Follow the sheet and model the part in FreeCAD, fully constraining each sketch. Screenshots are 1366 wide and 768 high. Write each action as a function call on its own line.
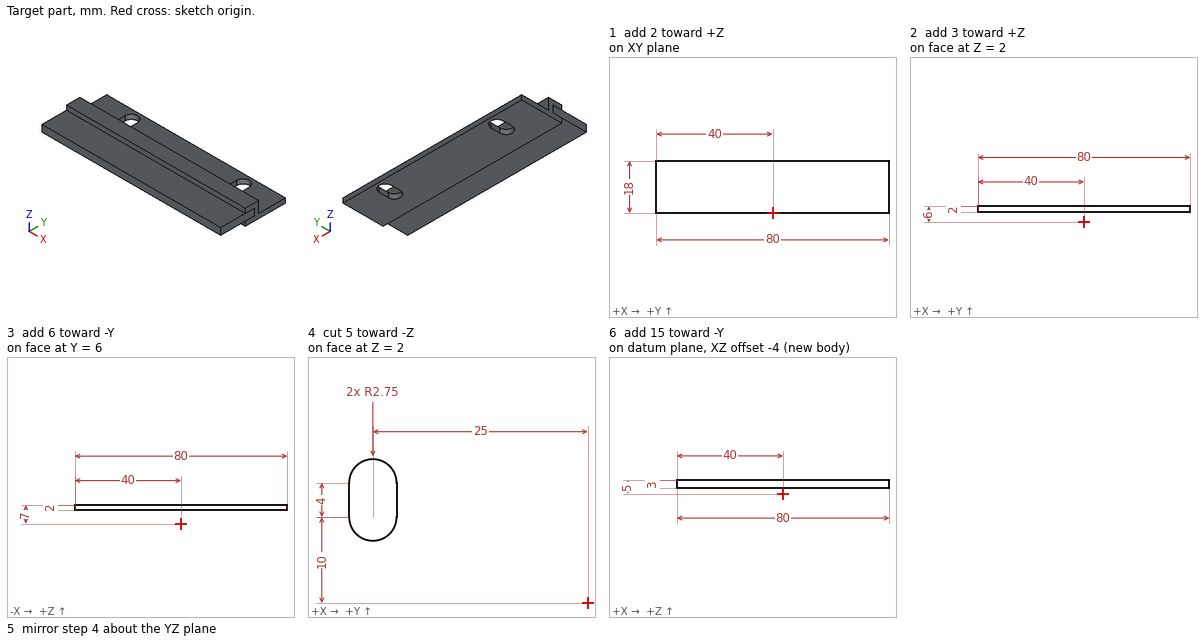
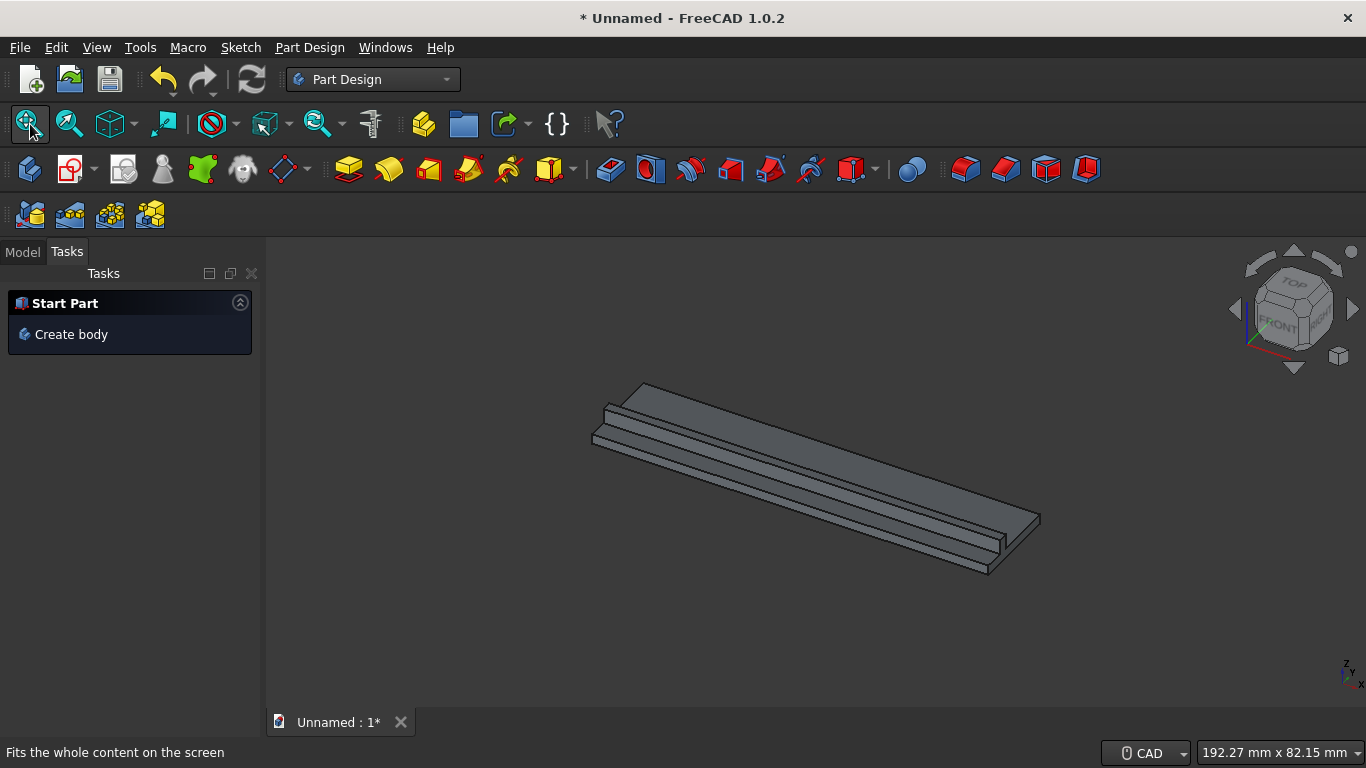
key(4)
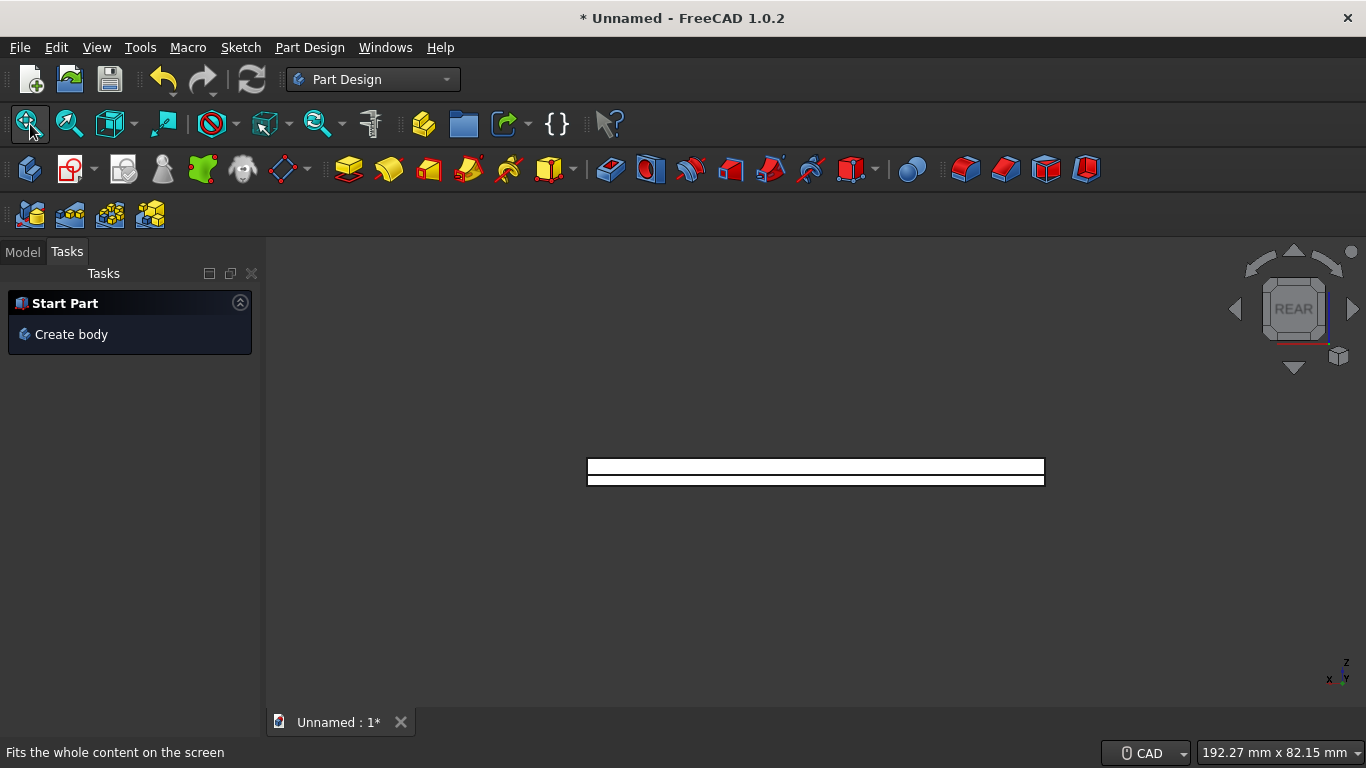
key(v)
key(f)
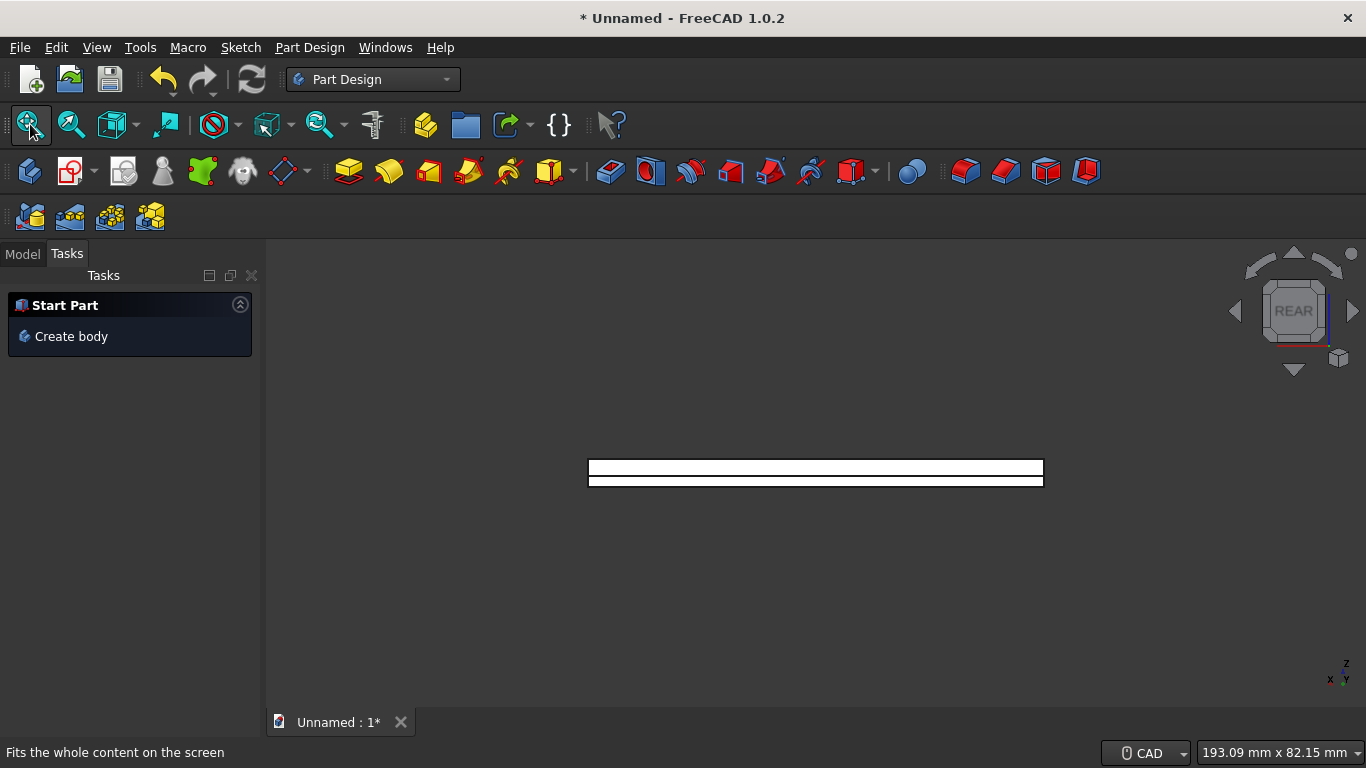
click(621, 466)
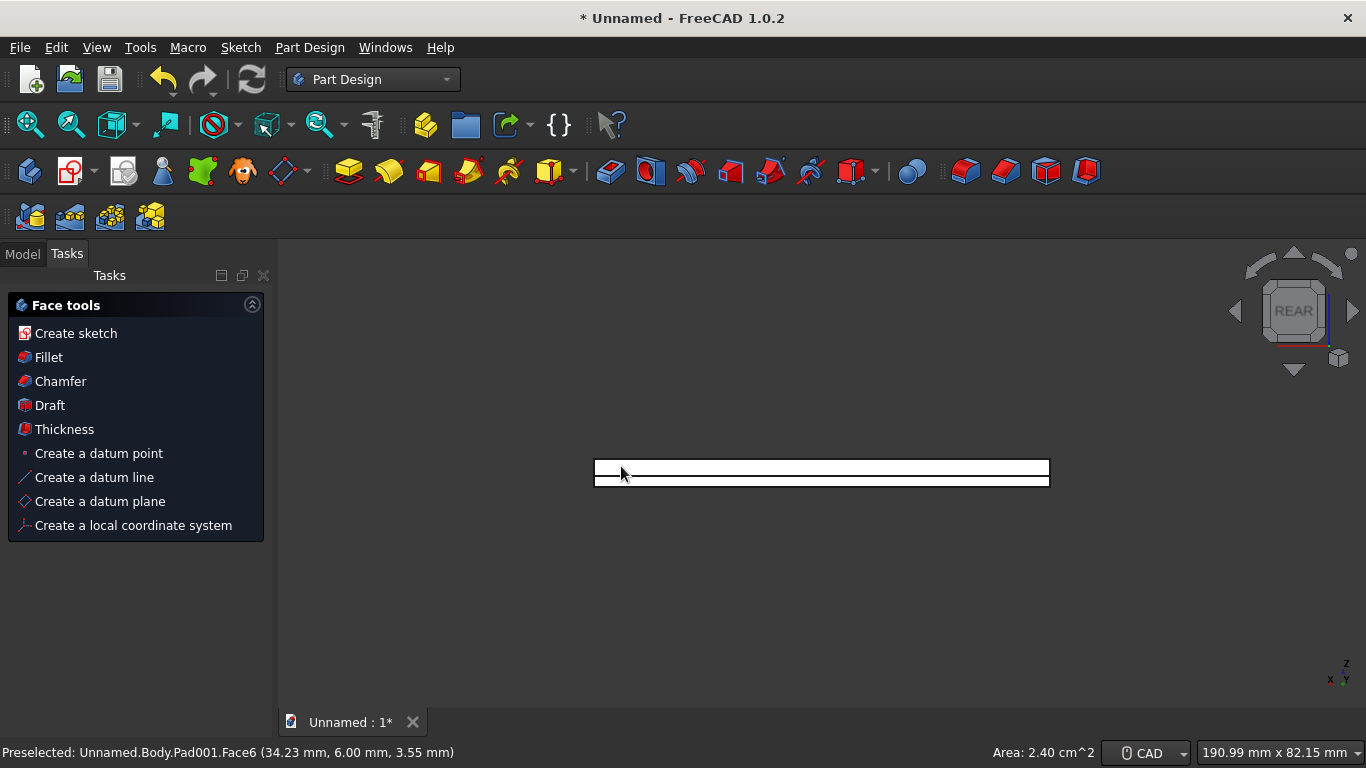
click(70, 172)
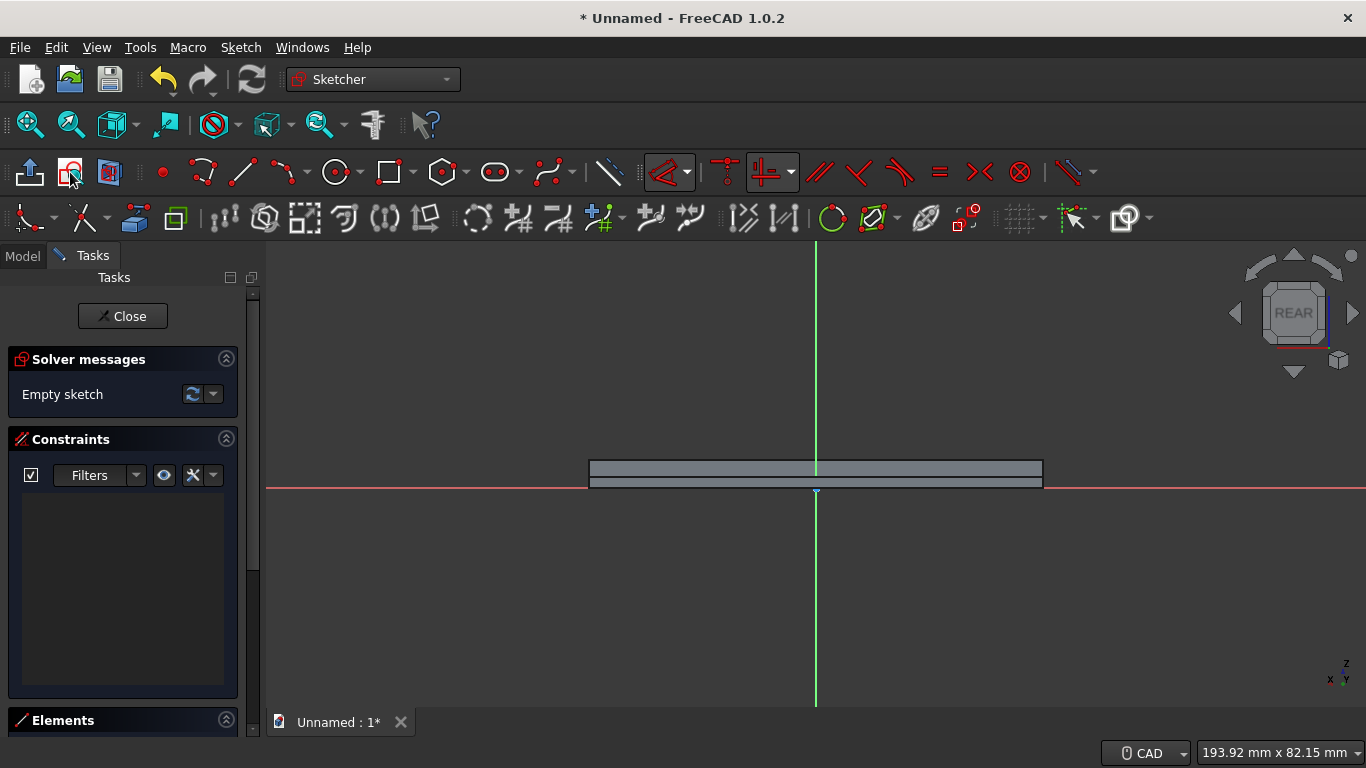
scroll(955, 457, up, 2)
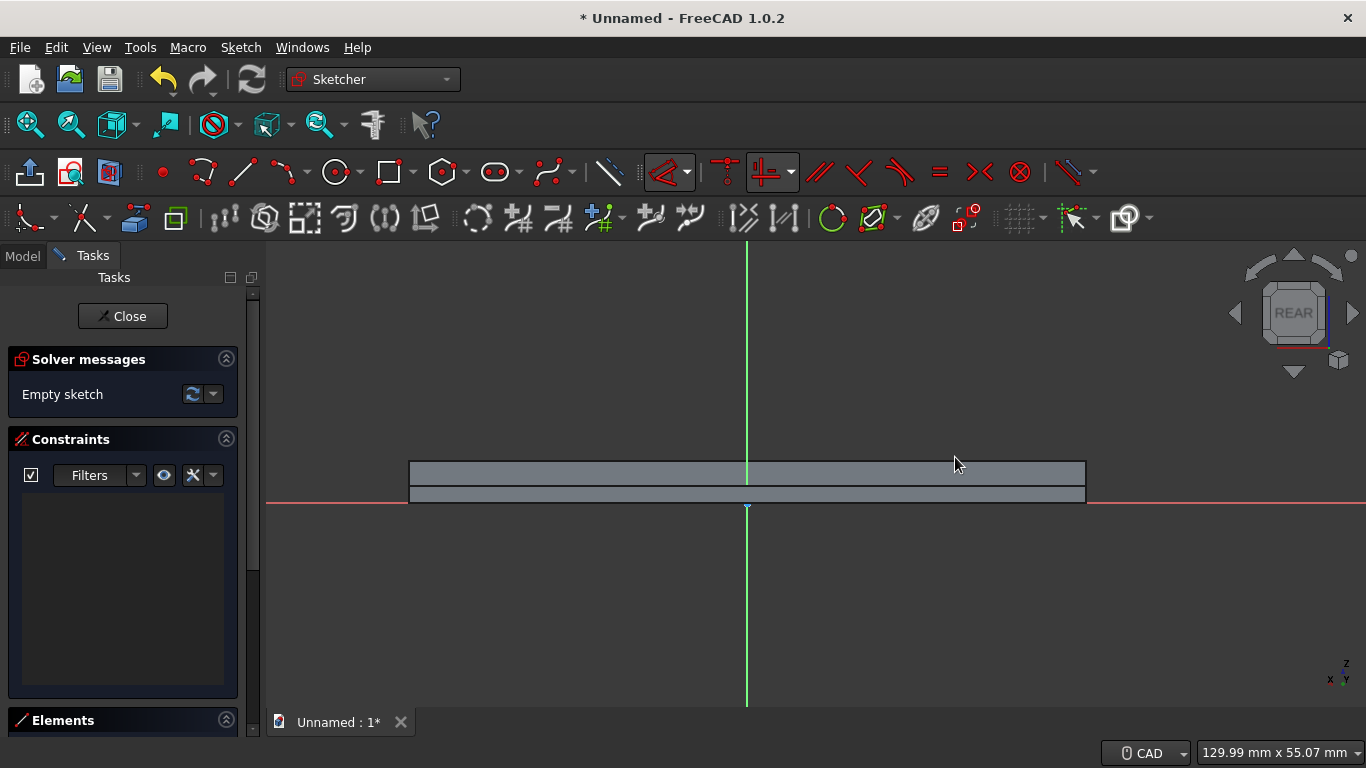
click(390, 172)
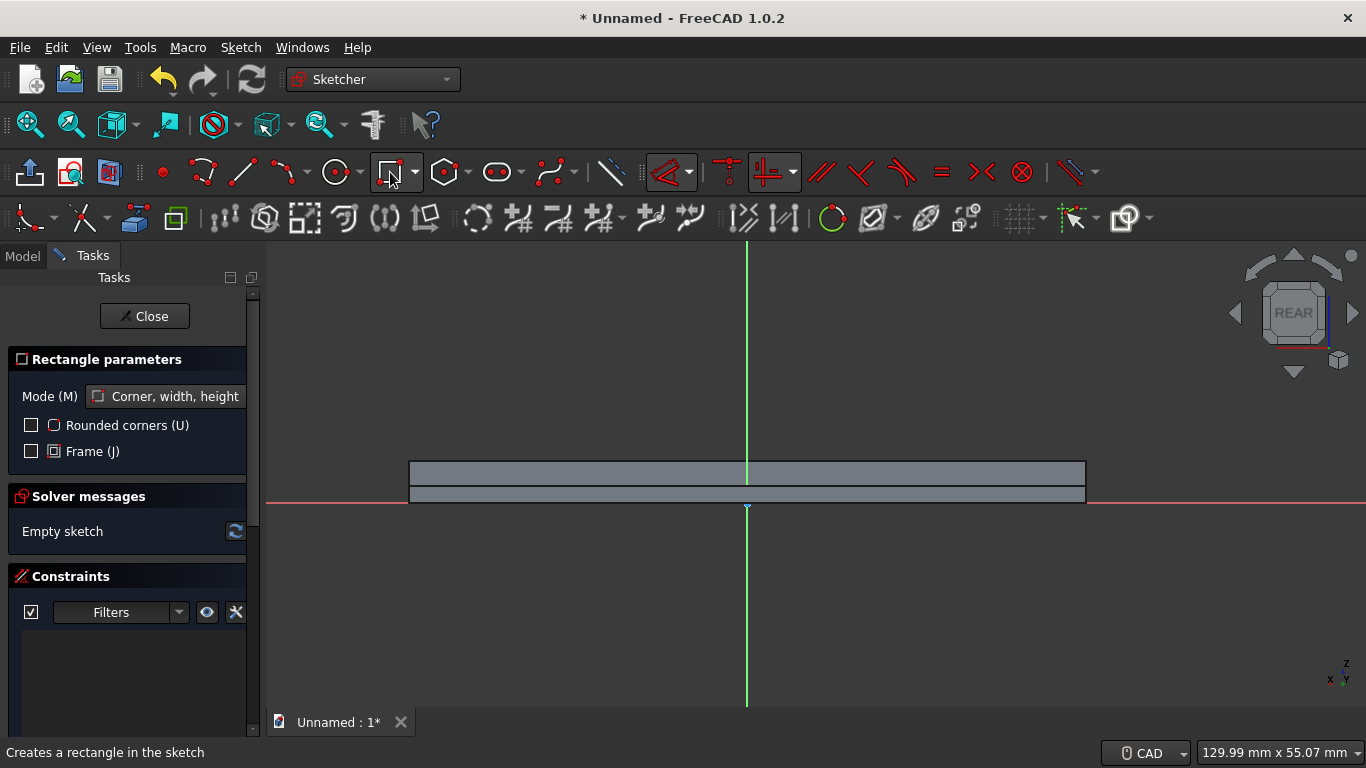
click(409, 444)
click(1086, 461)
key(Escape)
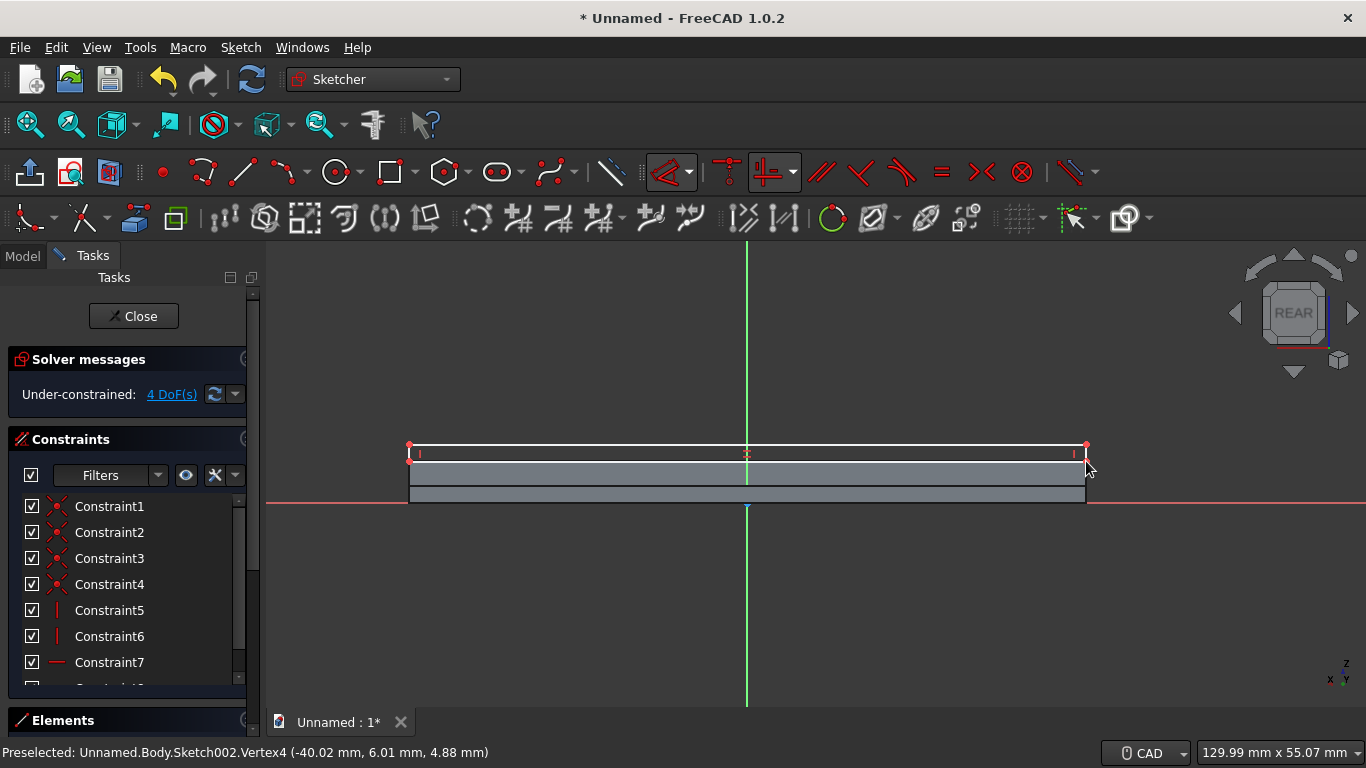
scroll(409, 454, up, 5)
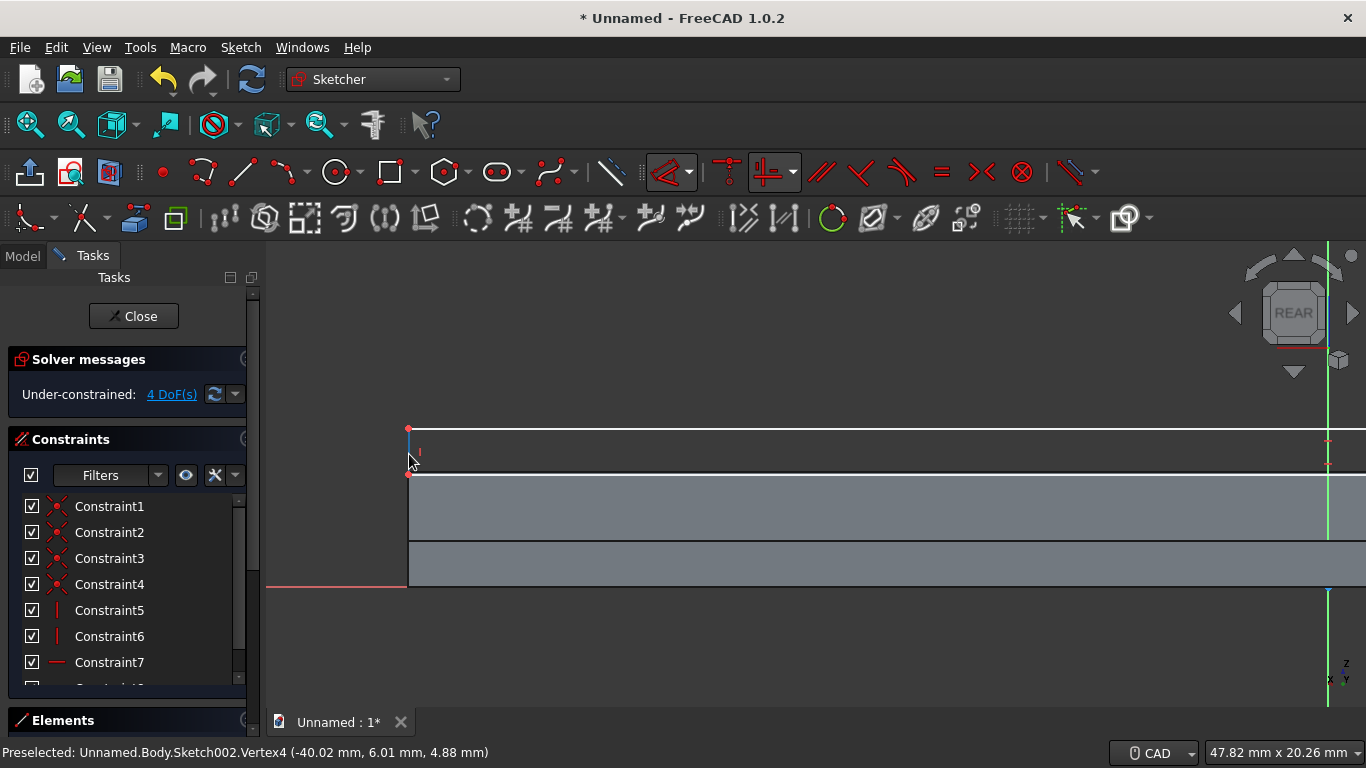
click(409, 452)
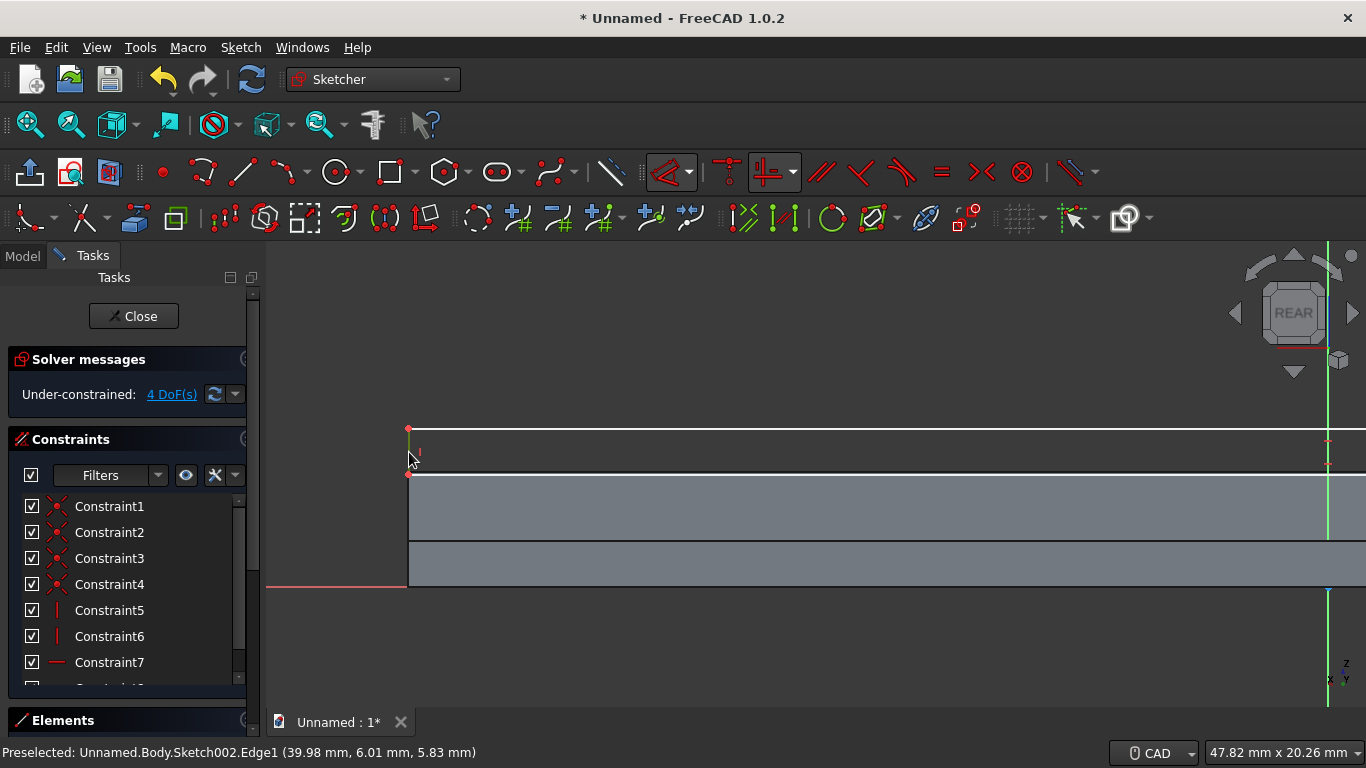
key(i)